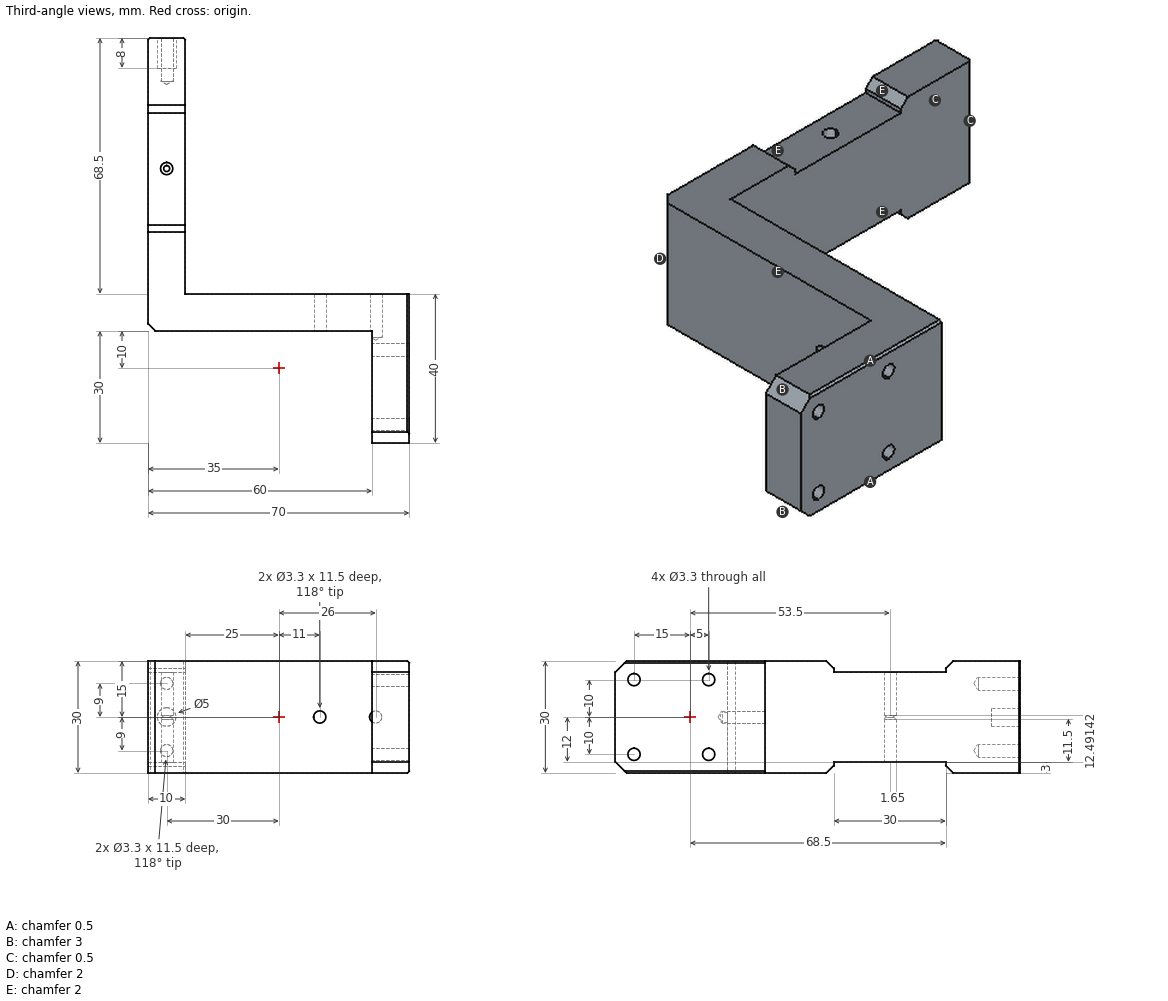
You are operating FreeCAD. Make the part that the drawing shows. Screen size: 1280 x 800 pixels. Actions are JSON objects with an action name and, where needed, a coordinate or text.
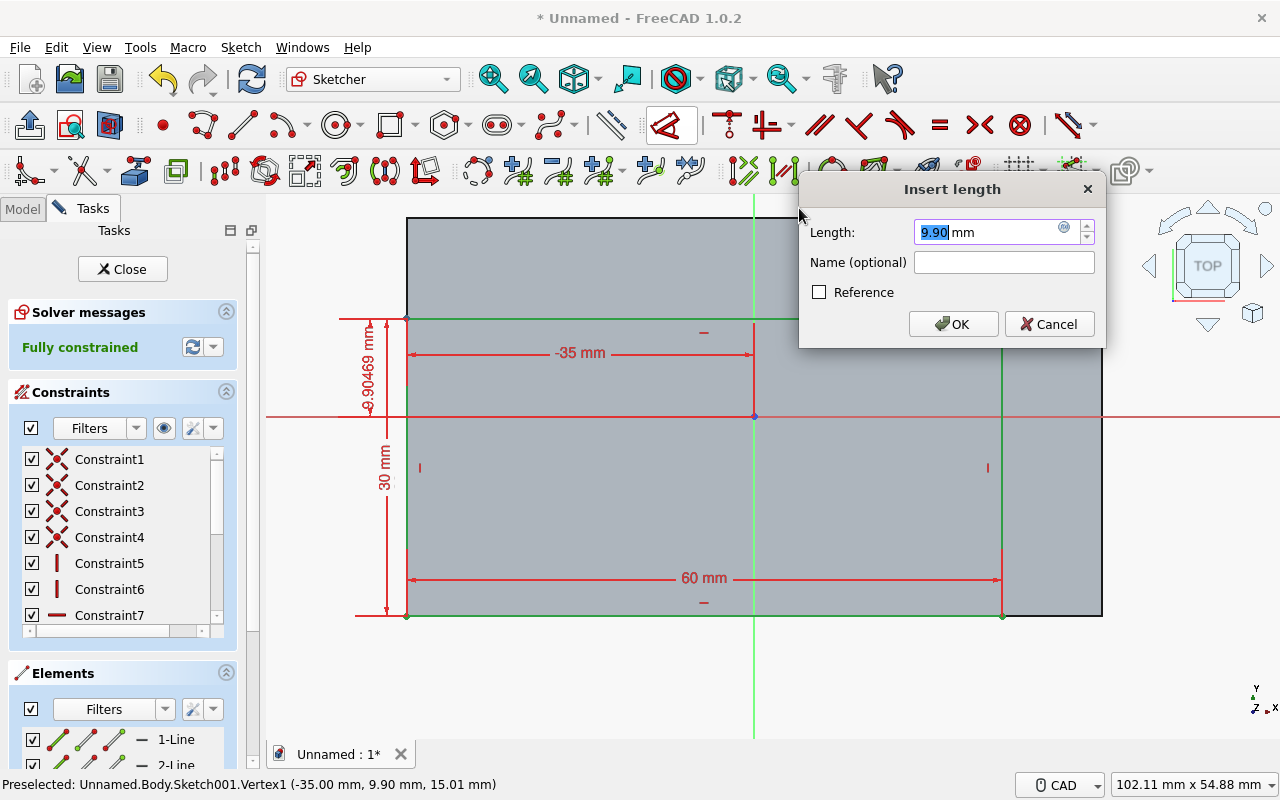
{"action": "type", "text": "10"}
{"action": "key", "text": "Return"}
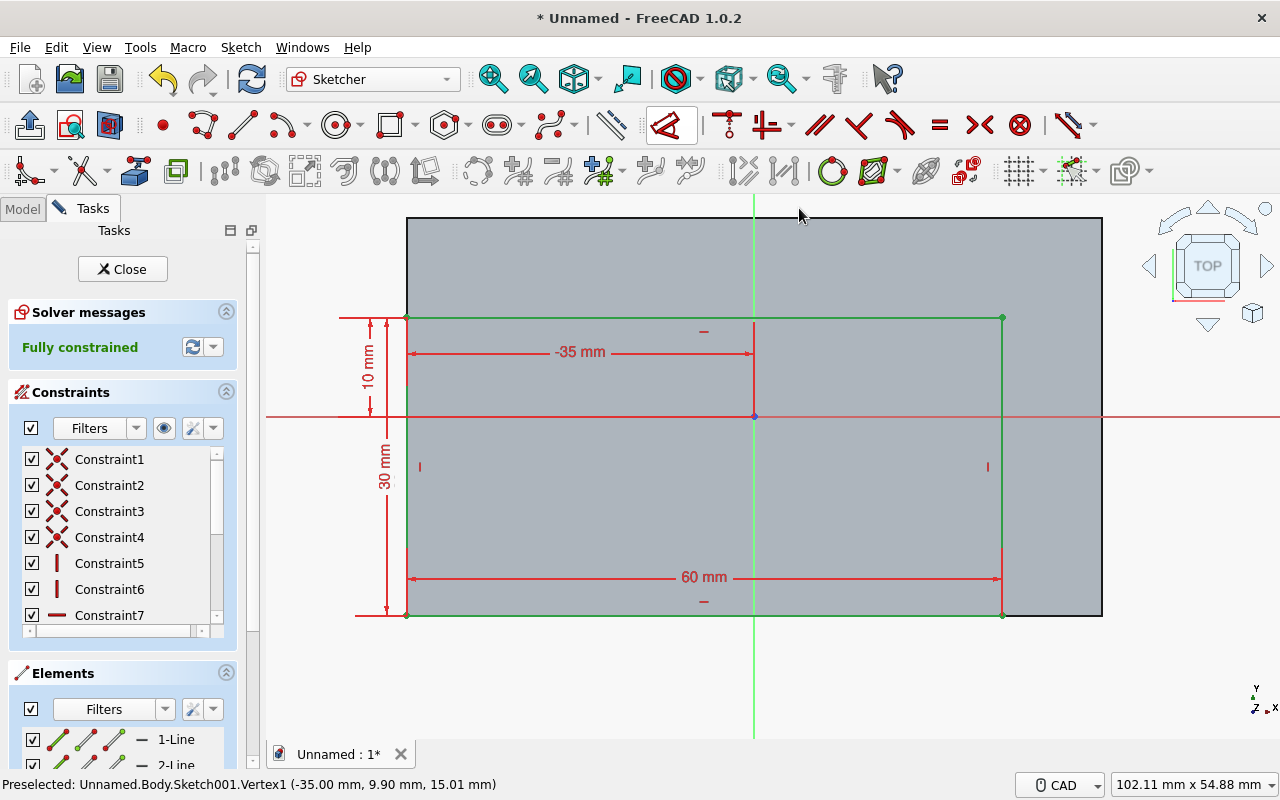
{"action": "left_click", "coordinate": [123, 269]}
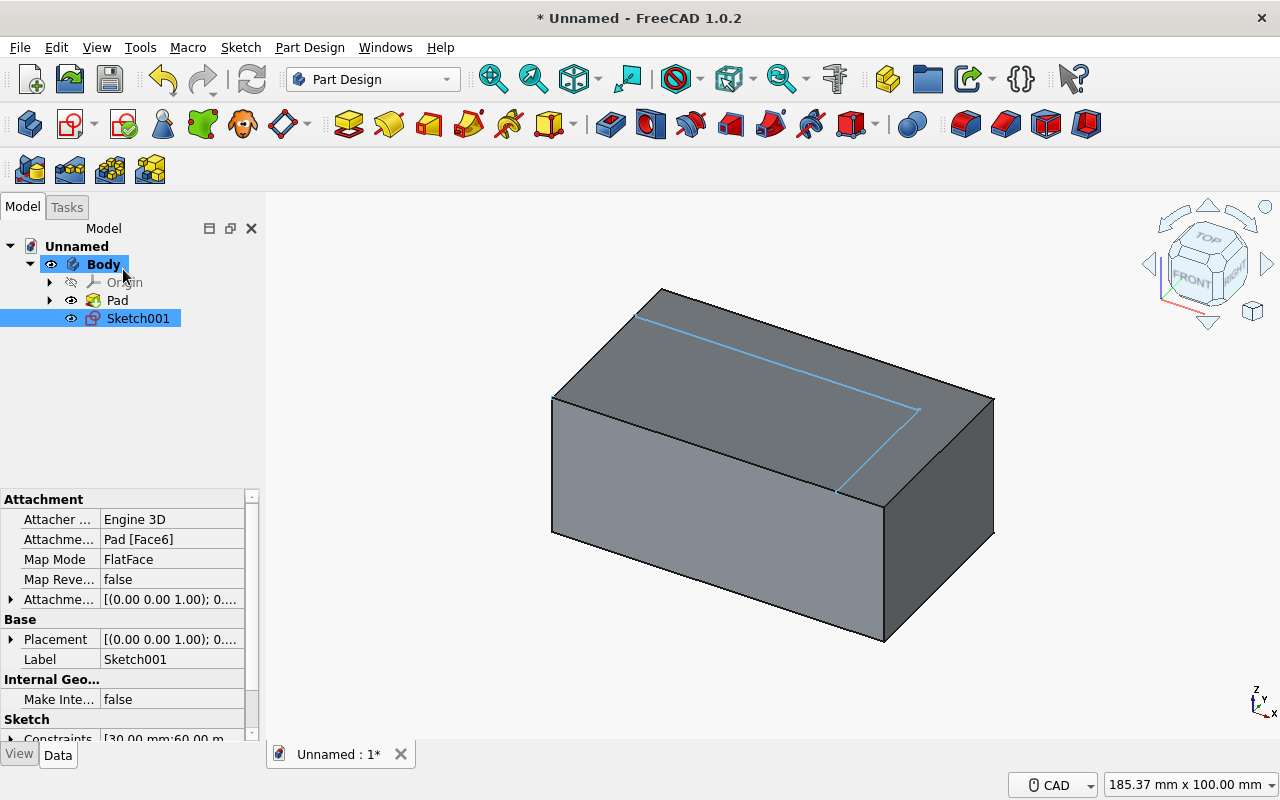
{"action": "left_click", "coordinate": [612, 124]}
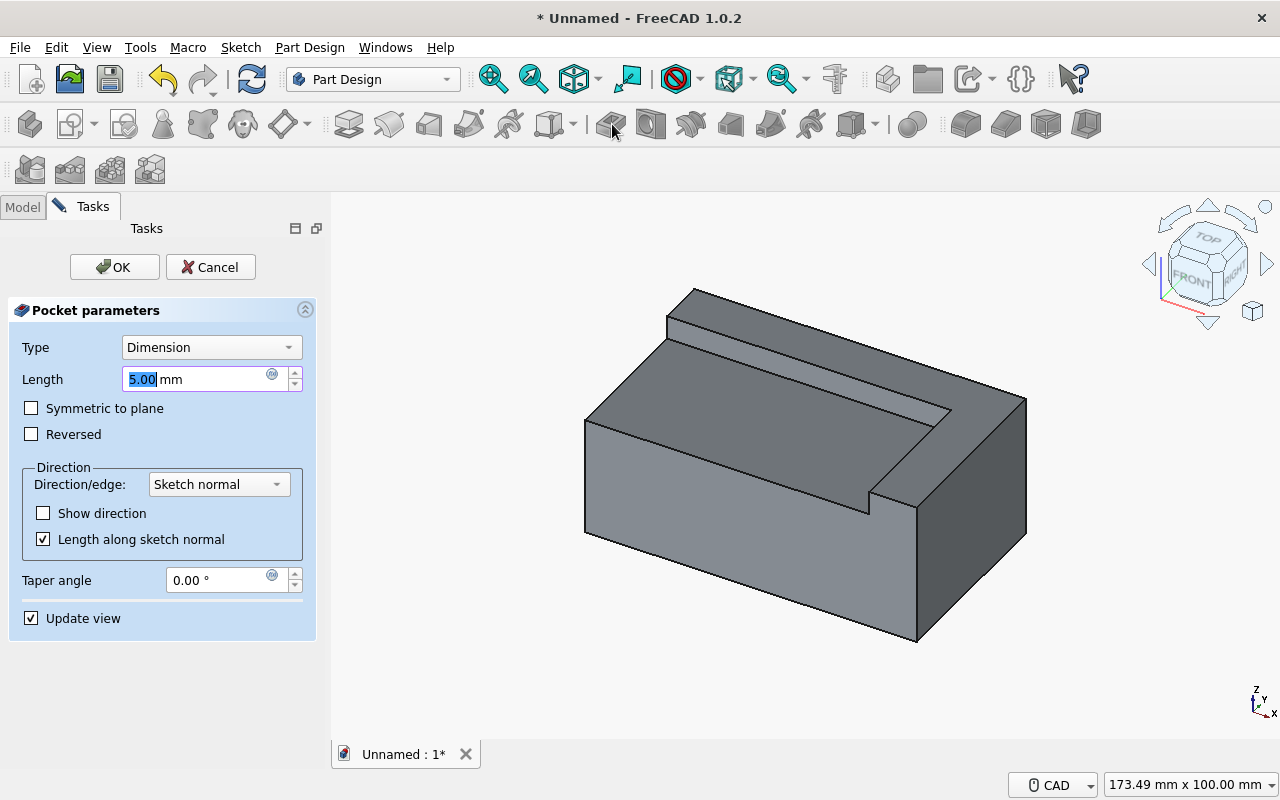
{"action": "left_click", "coordinate": [212, 348]}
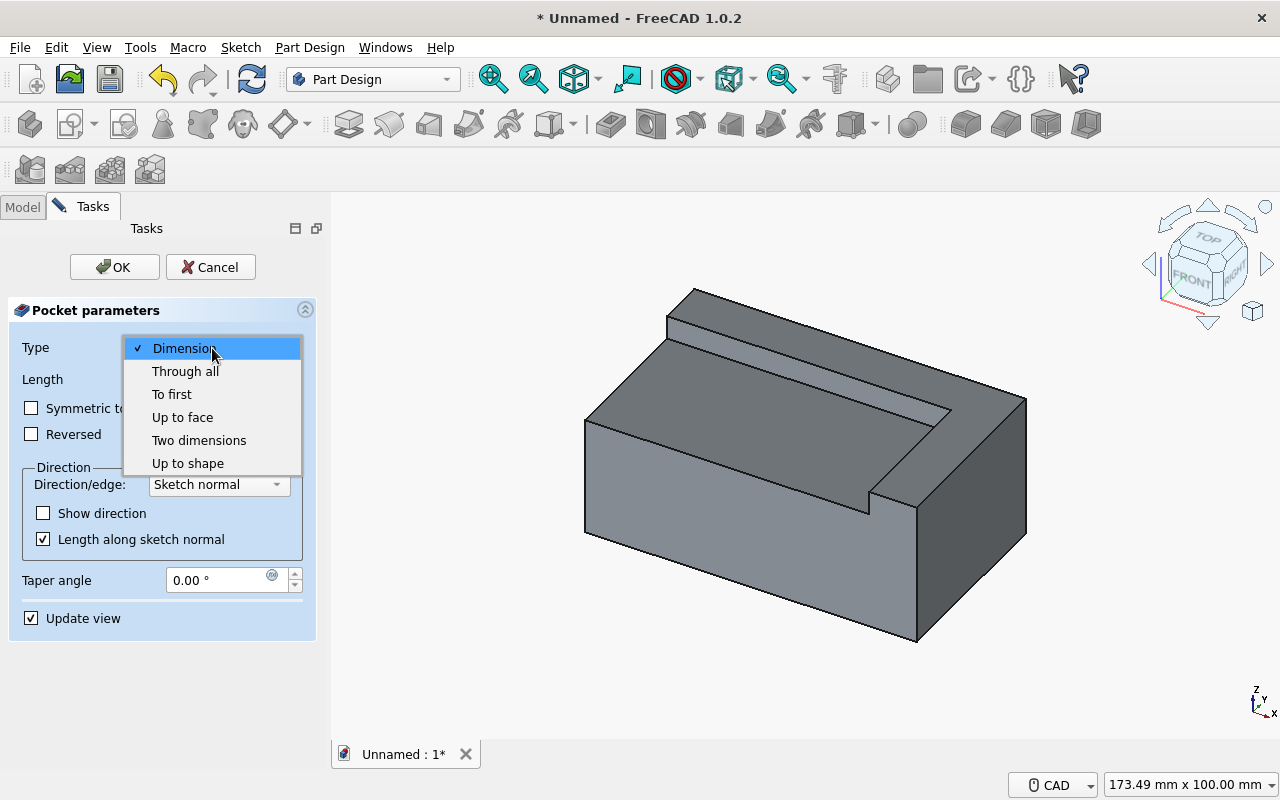
{"action": "left_click", "coordinate": [212, 372]}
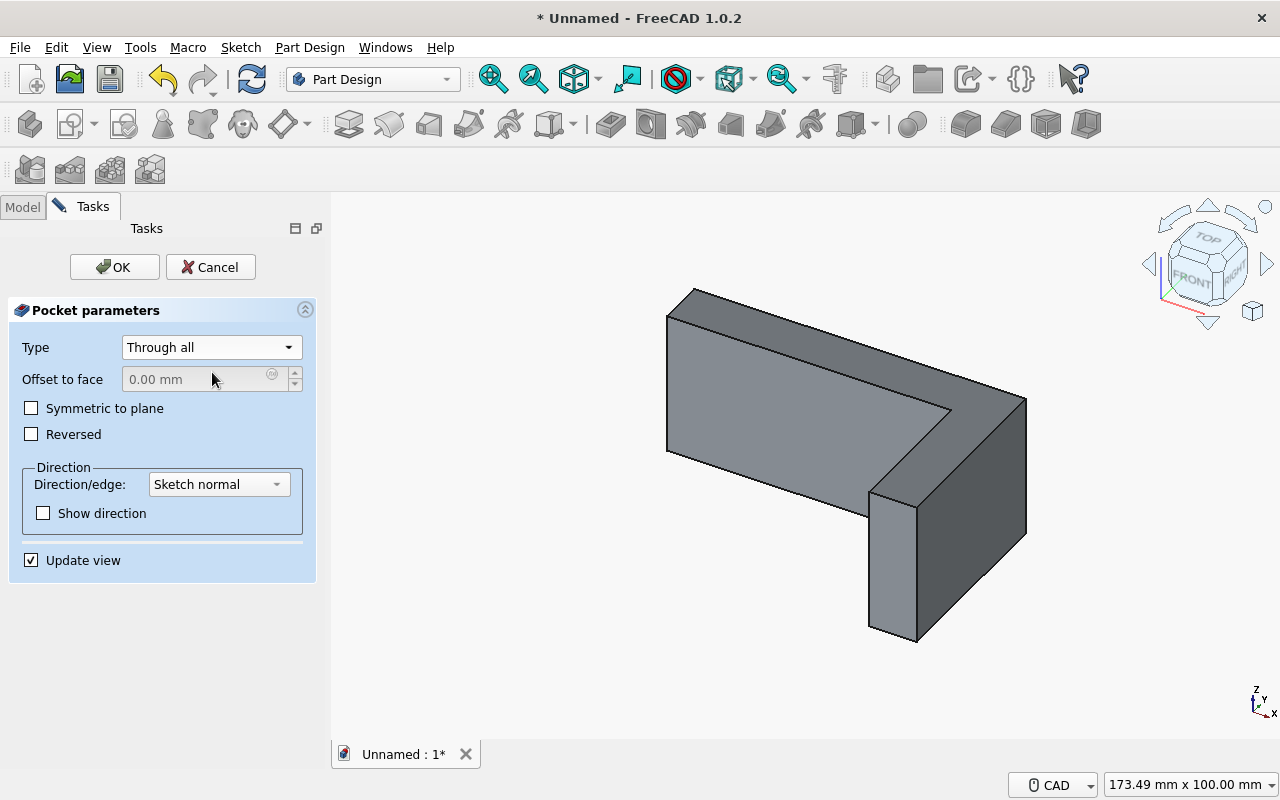
{"action": "left_click", "coordinate": [115, 267]}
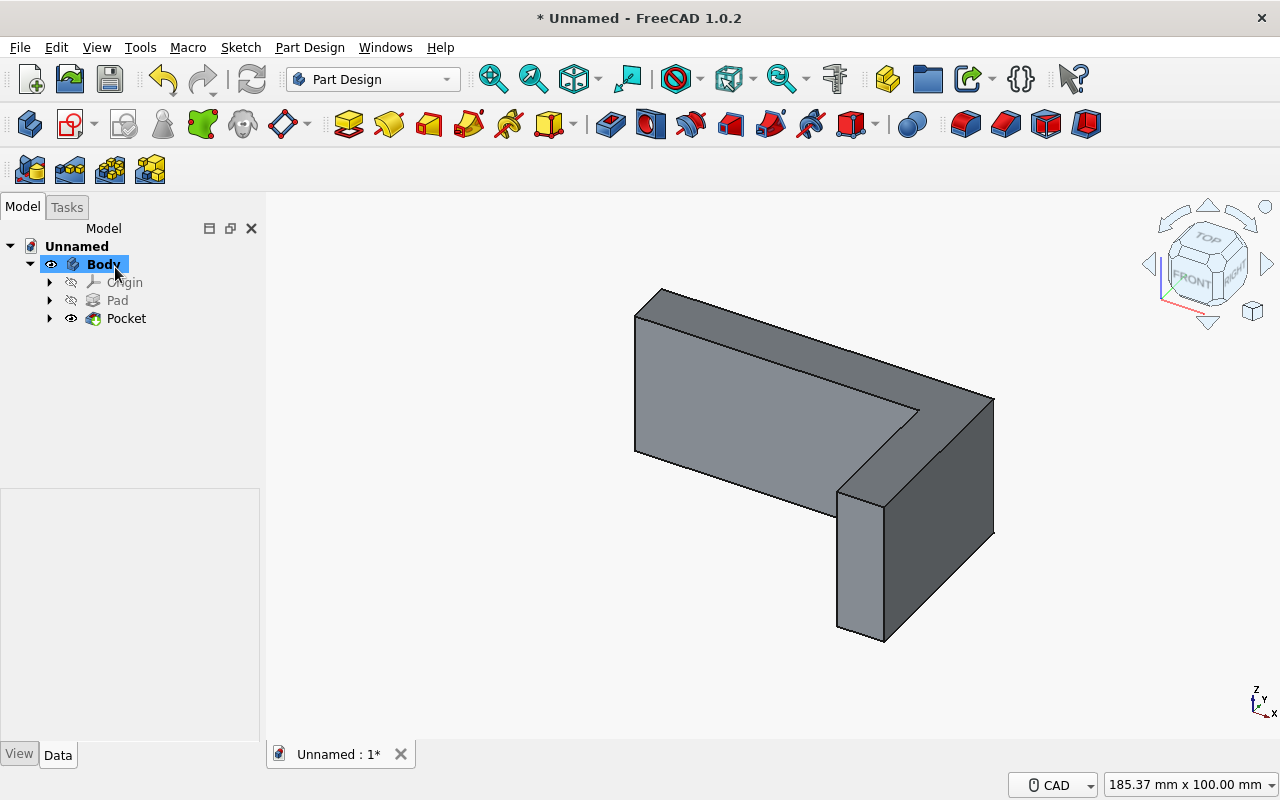
{"action": "left_click", "coordinate": [939, 452]}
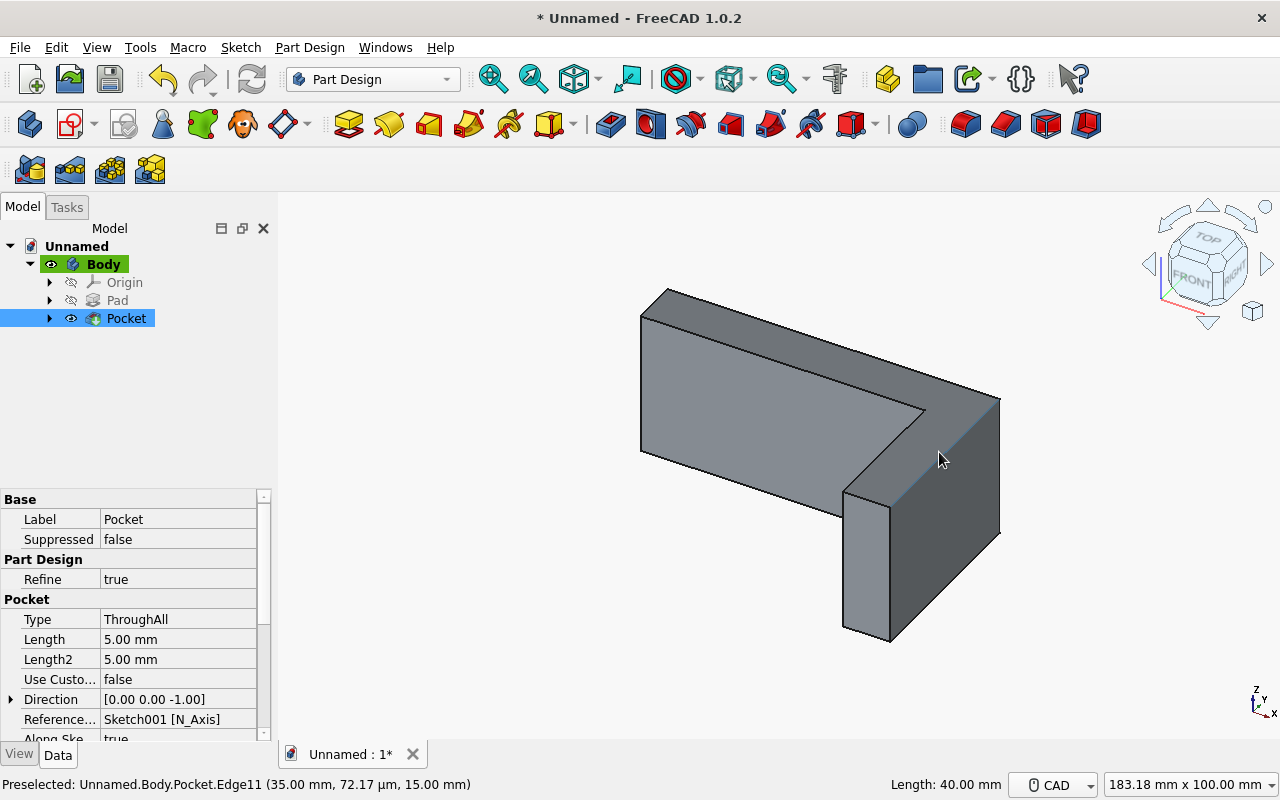
{"action": "key", "text": "0"}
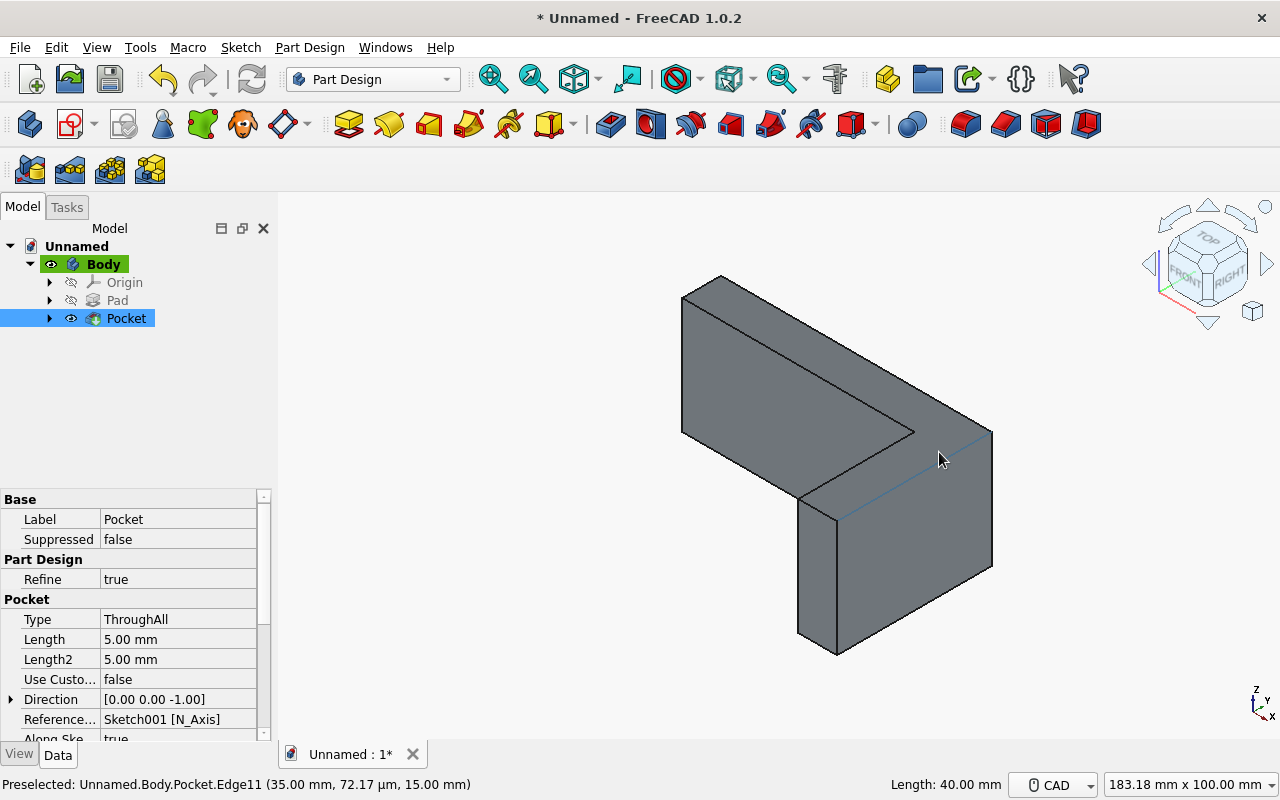
{"action": "key", "text": "2"}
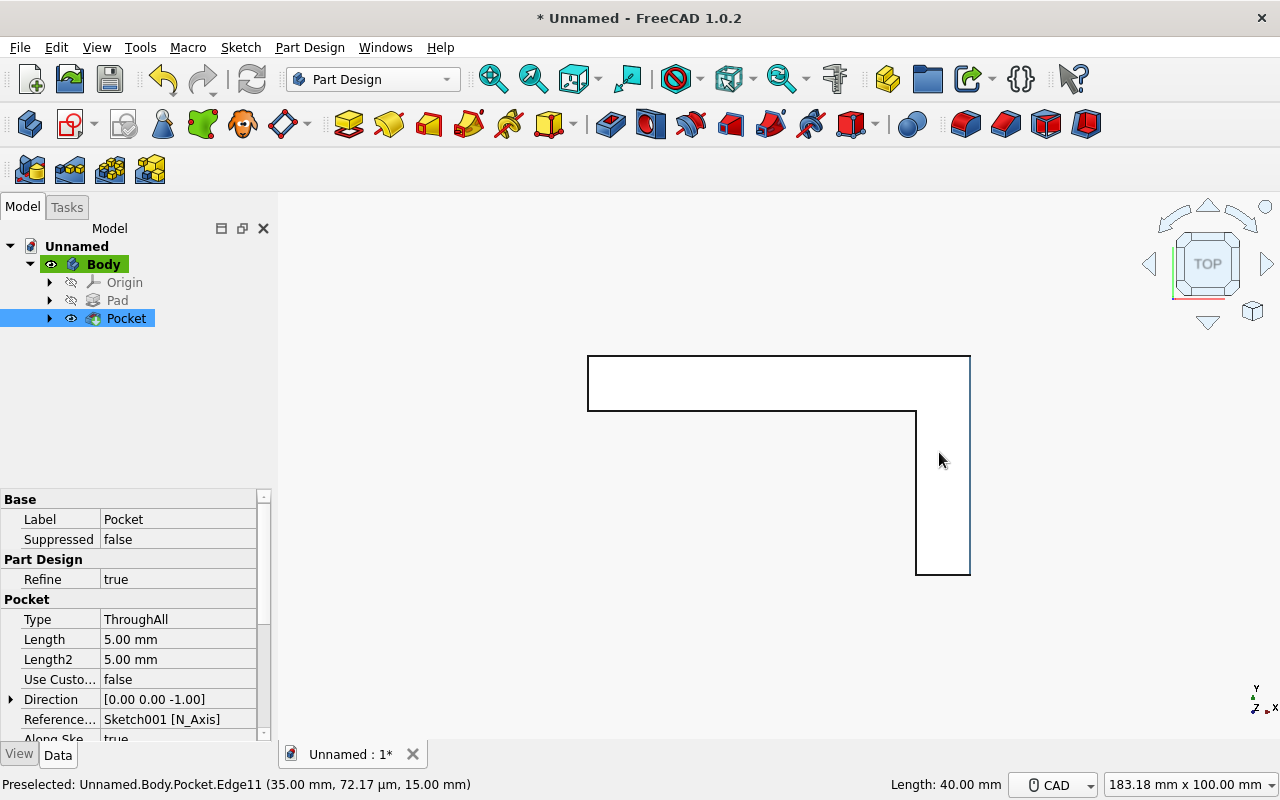
{"action": "left_click", "coordinate": [494, 80]}